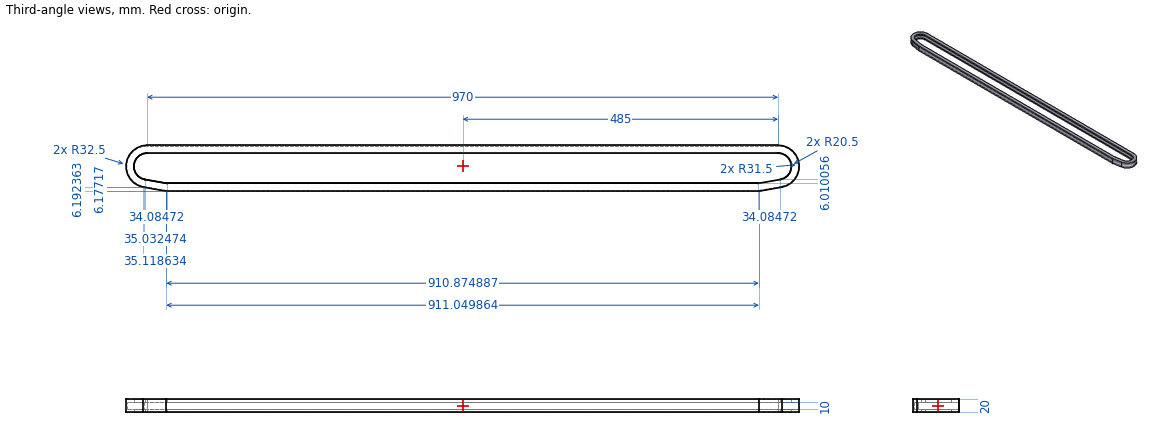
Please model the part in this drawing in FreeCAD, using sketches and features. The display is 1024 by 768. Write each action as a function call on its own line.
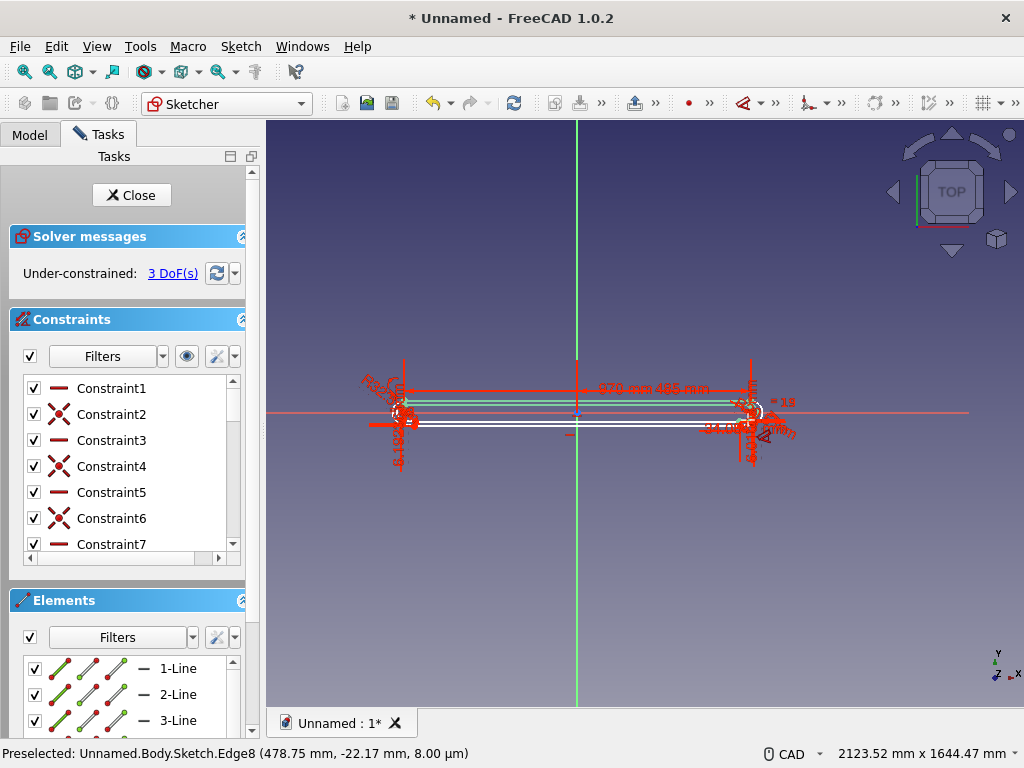
scroll(412, 421, up, 7)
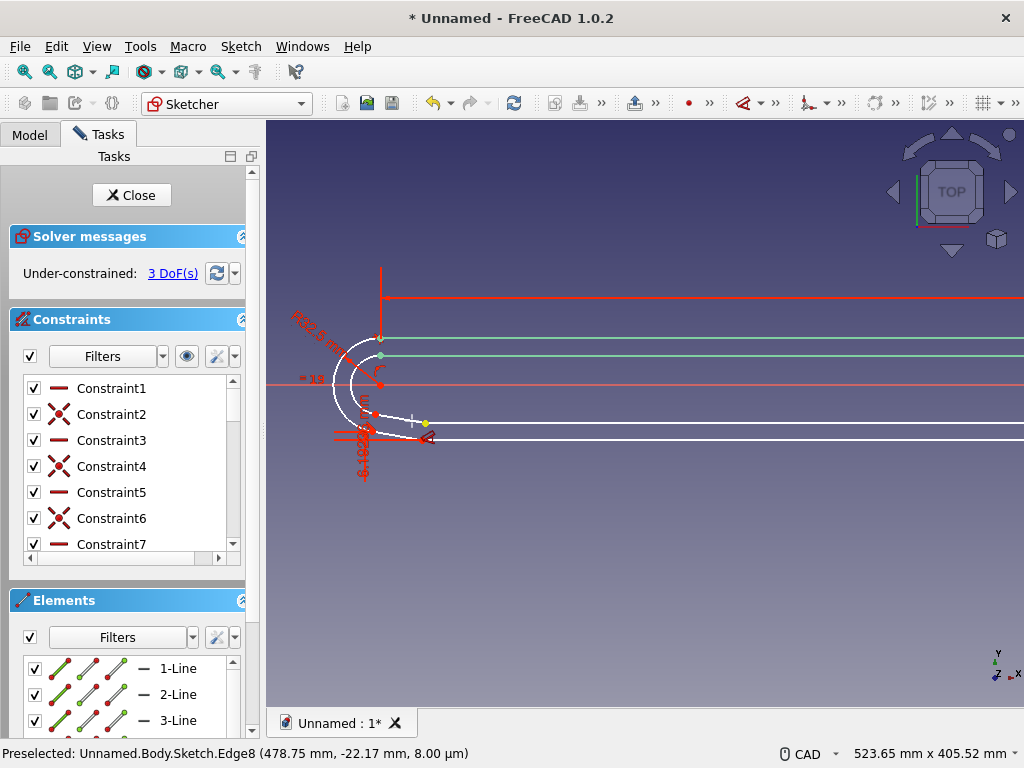
click(410, 421)
click(400, 457)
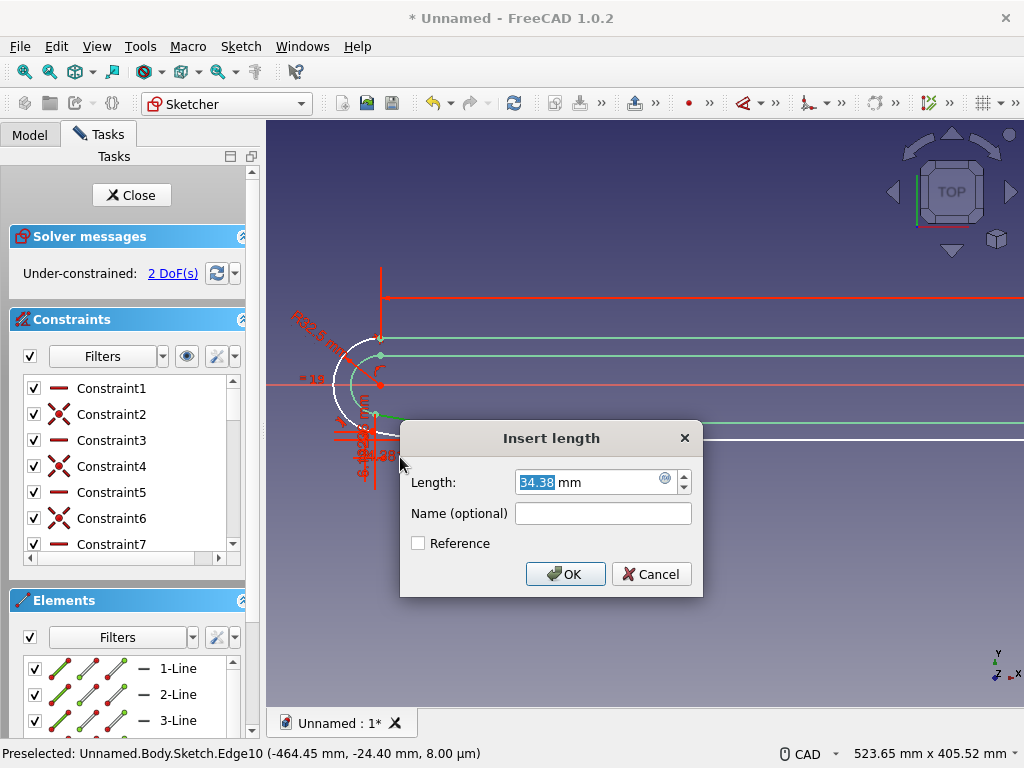
text(34.08472)
key(Return)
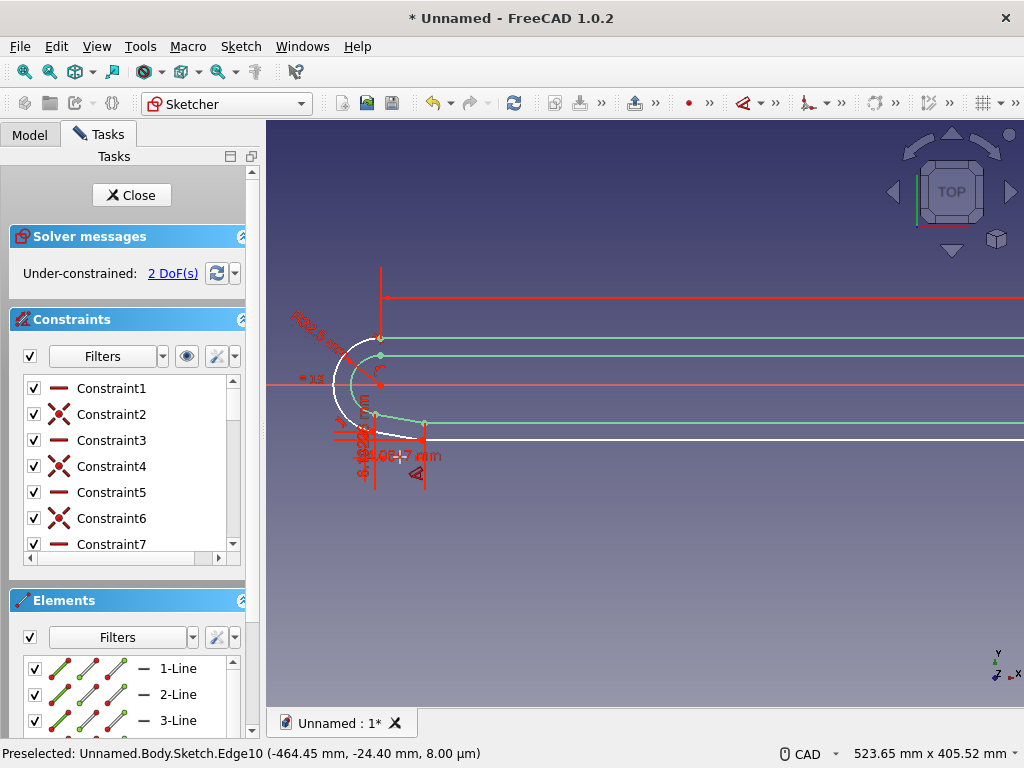
click(818, 440)
click(641, 474)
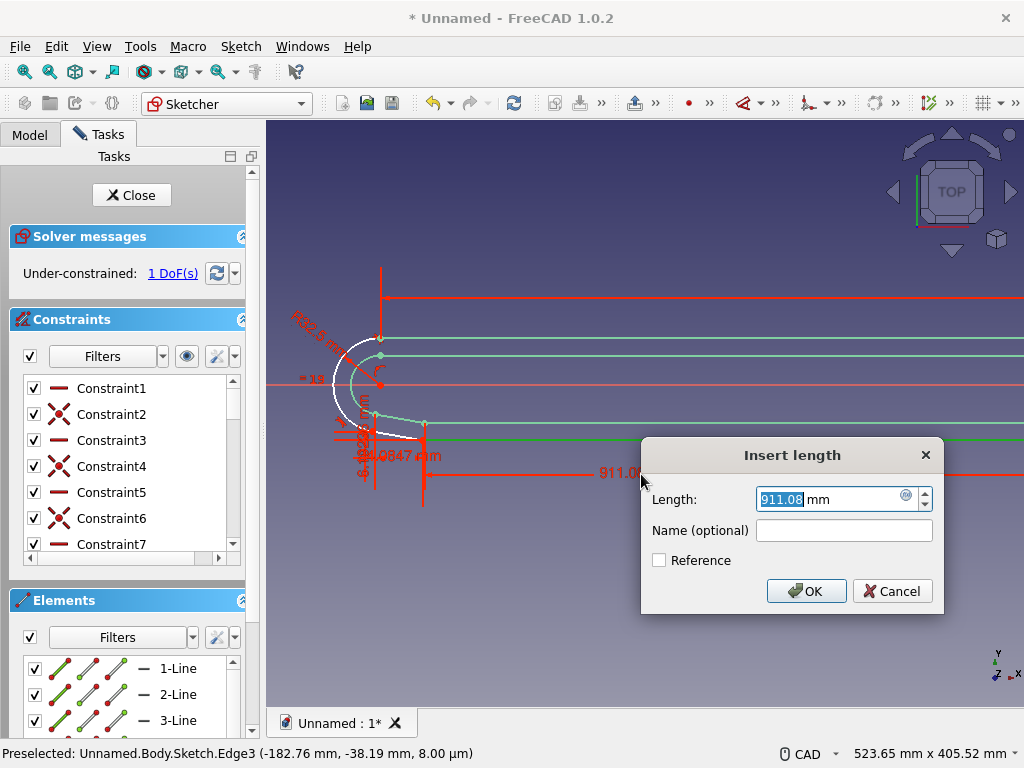
text(911.049864)
key(Return)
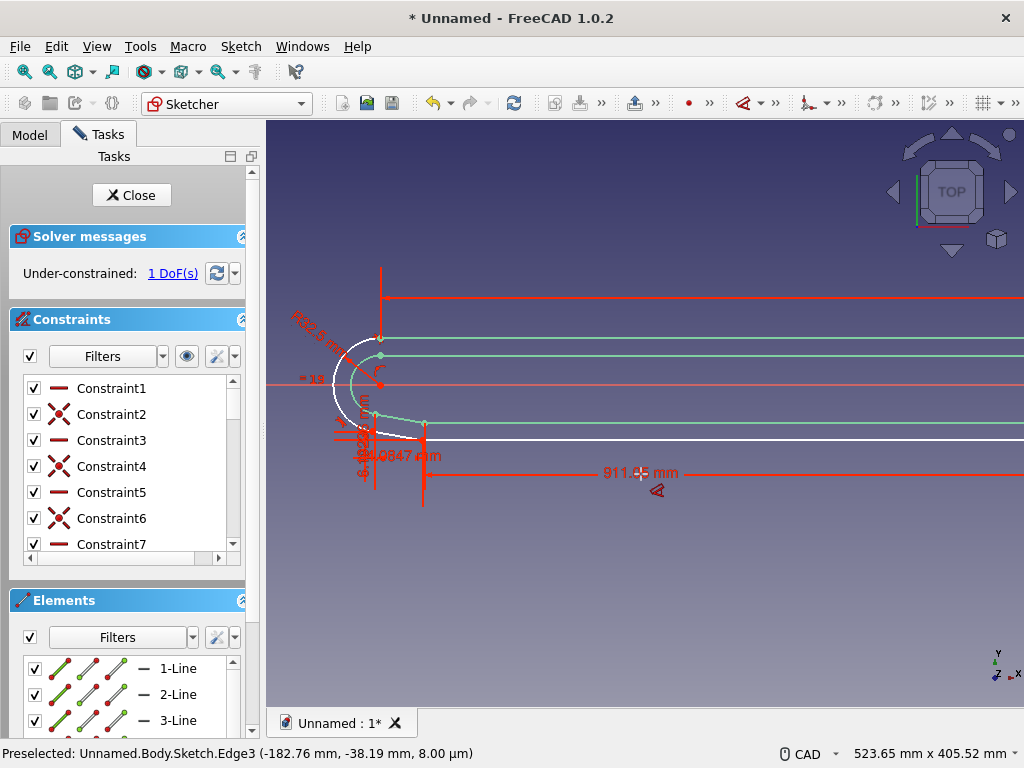
click(387, 434)
click(398, 498)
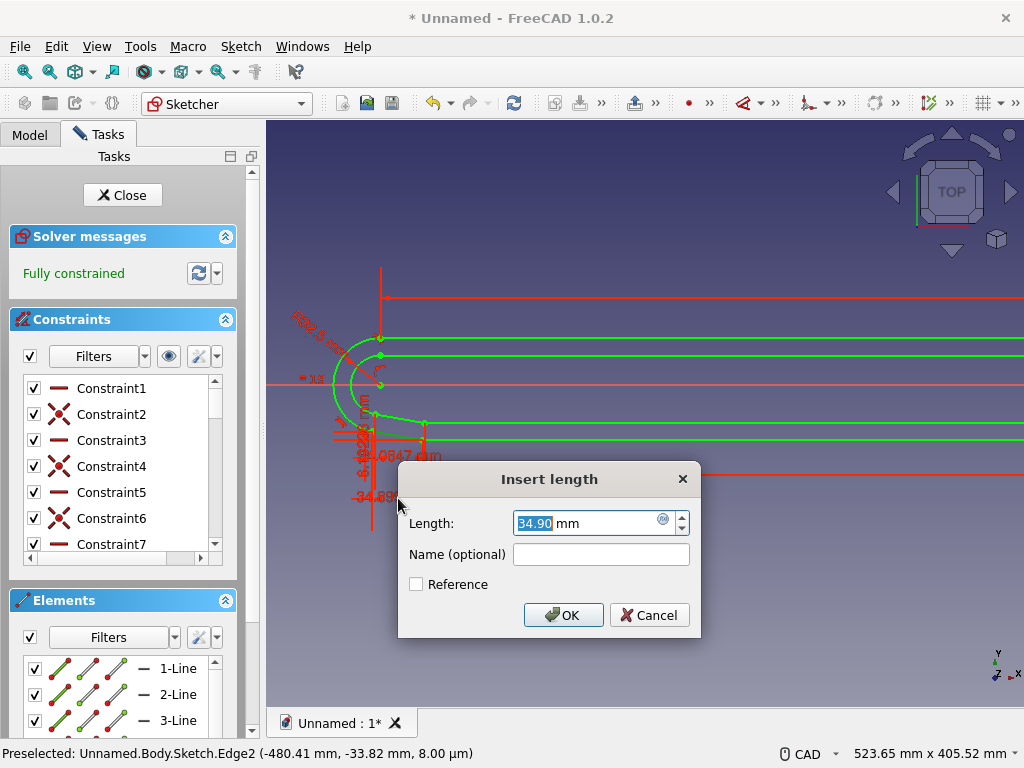
text(35.118634)
key(Return)
key(Escape)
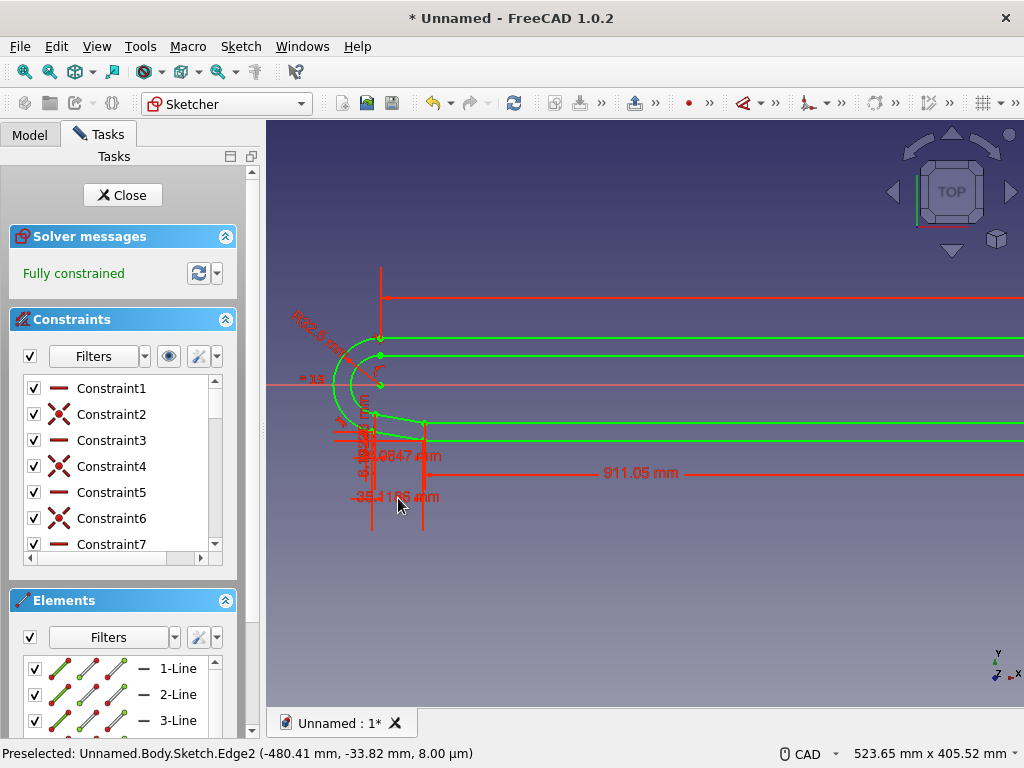
click(123, 195)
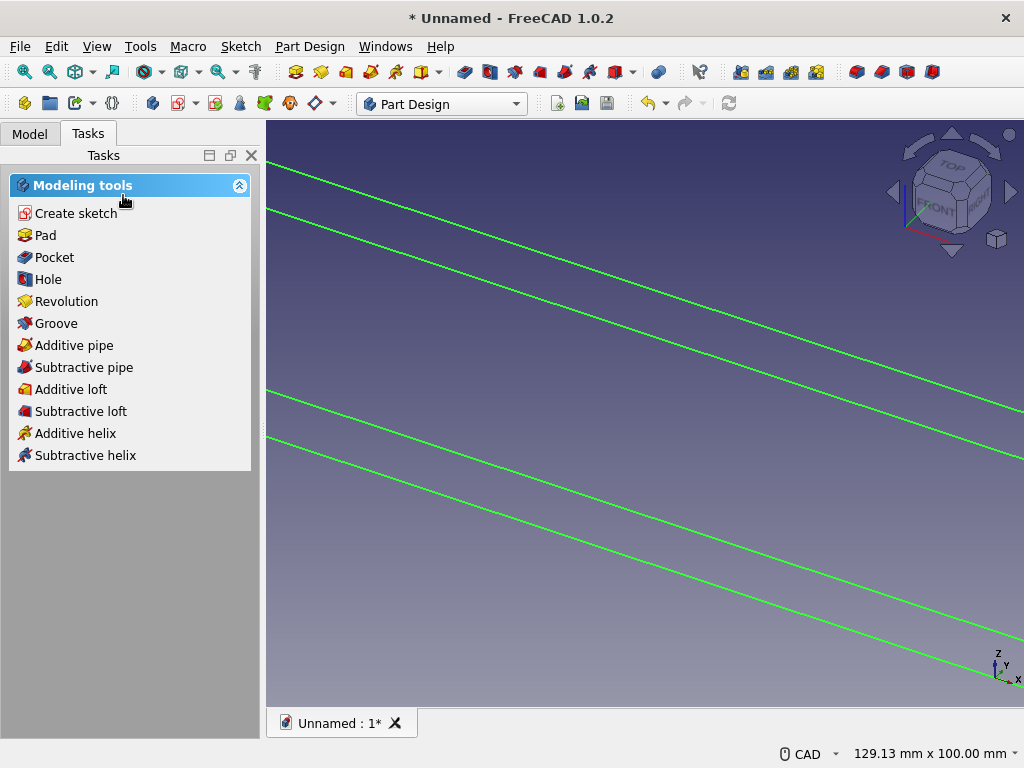
click(296, 72)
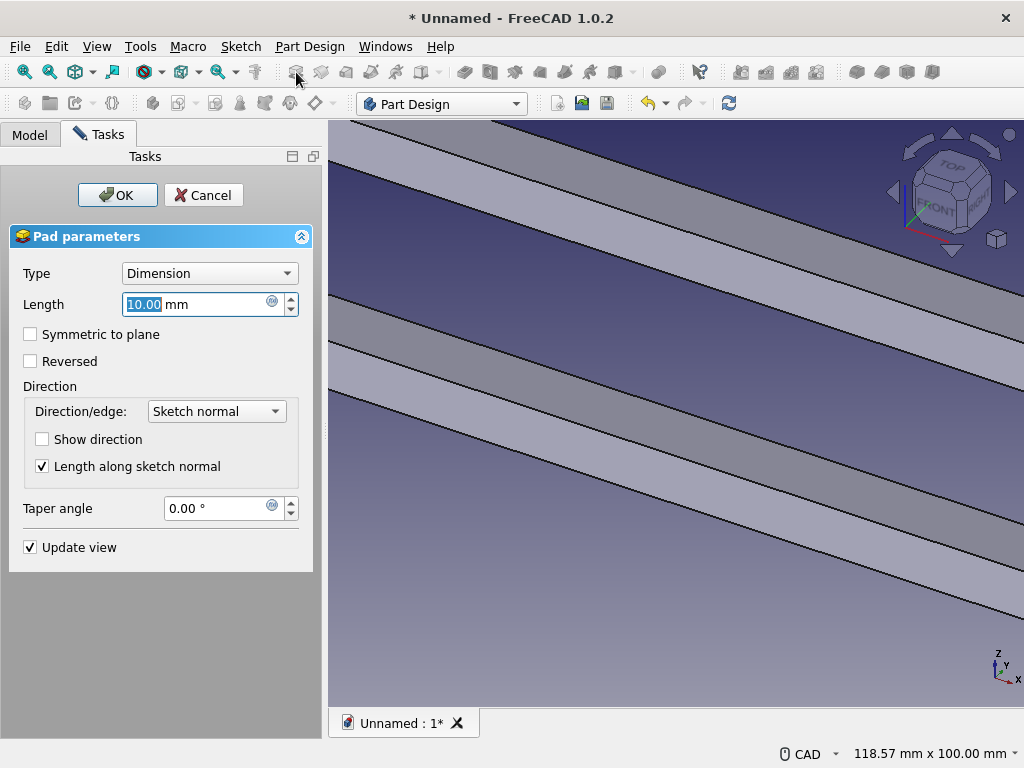
text(20)
key(Tab)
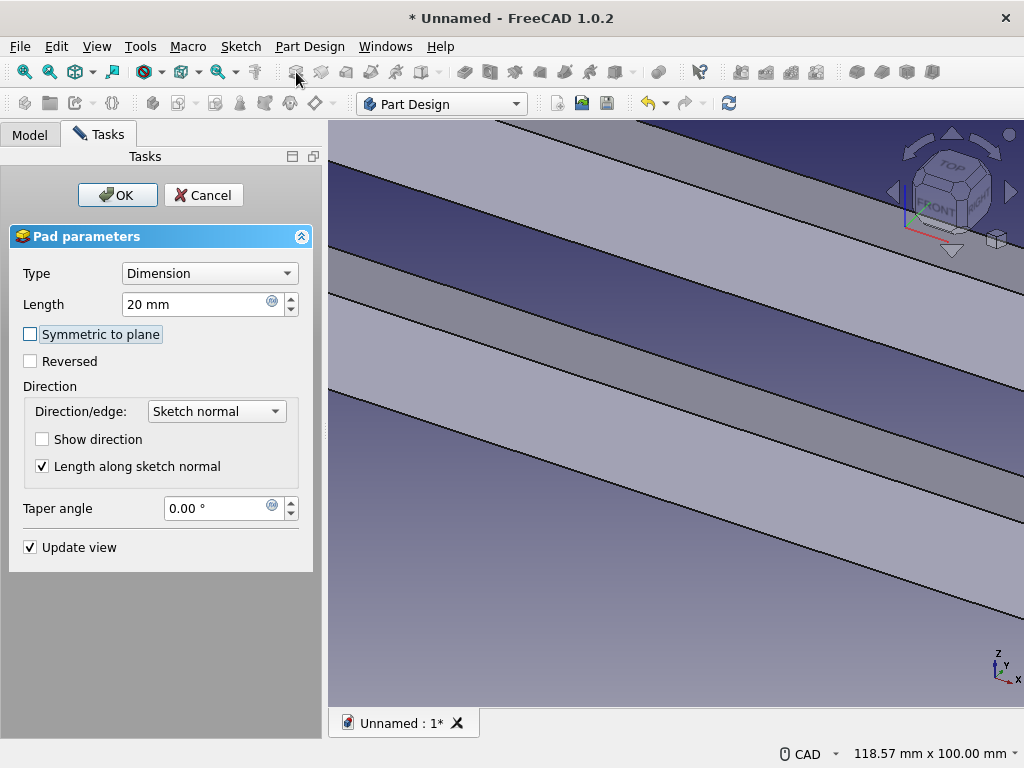
click(31, 334)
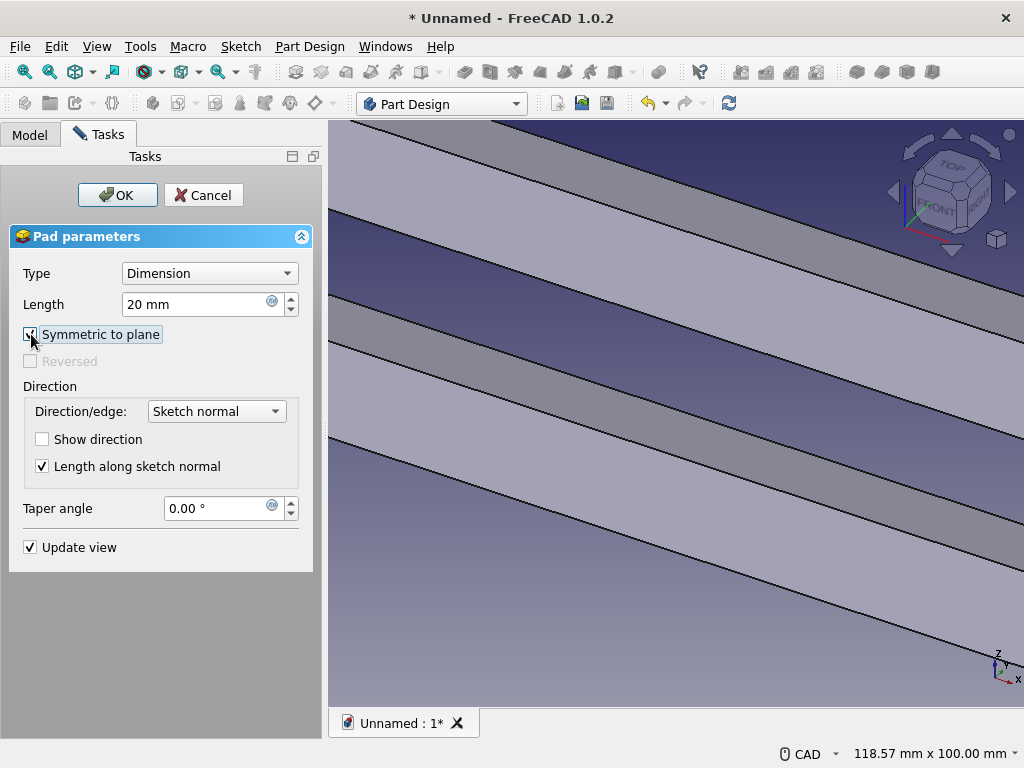
click(118, 195)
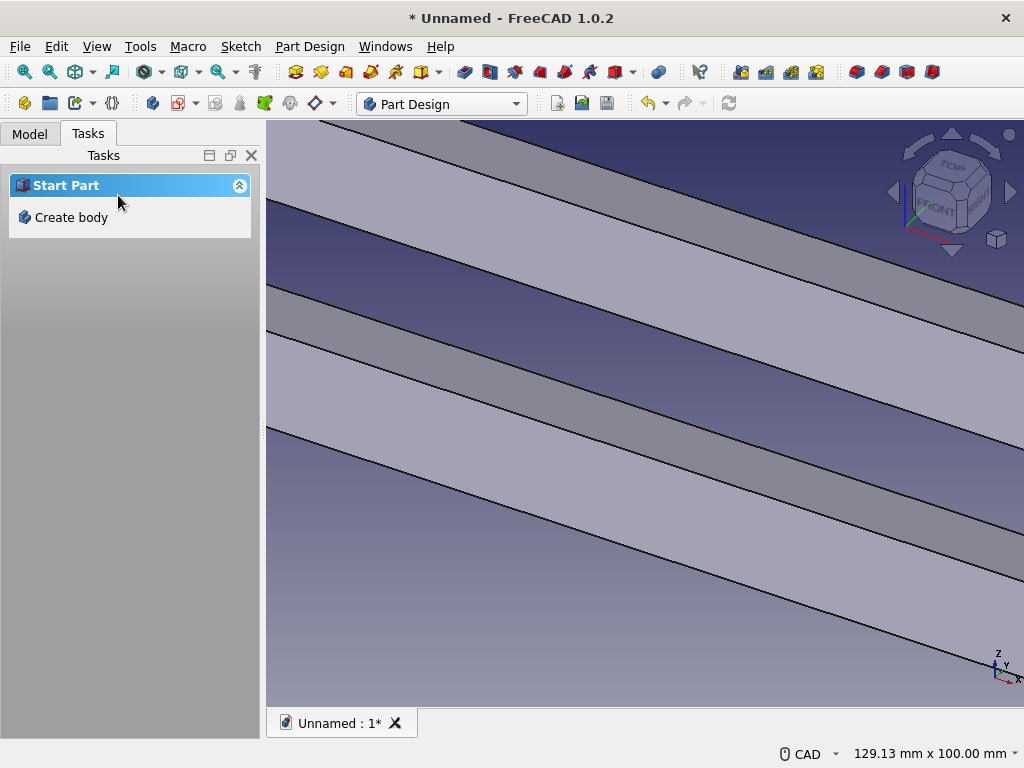
key(v)
key(f)